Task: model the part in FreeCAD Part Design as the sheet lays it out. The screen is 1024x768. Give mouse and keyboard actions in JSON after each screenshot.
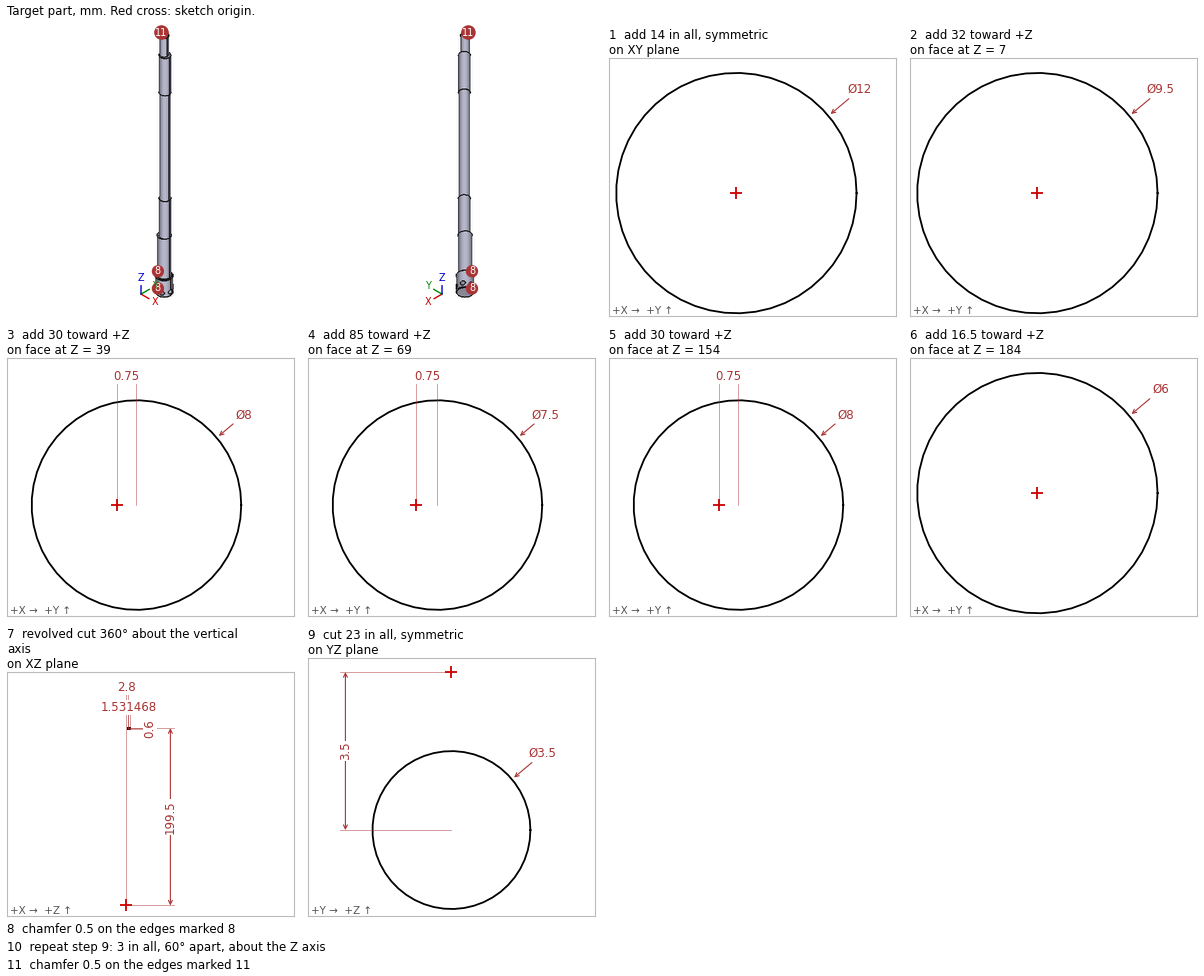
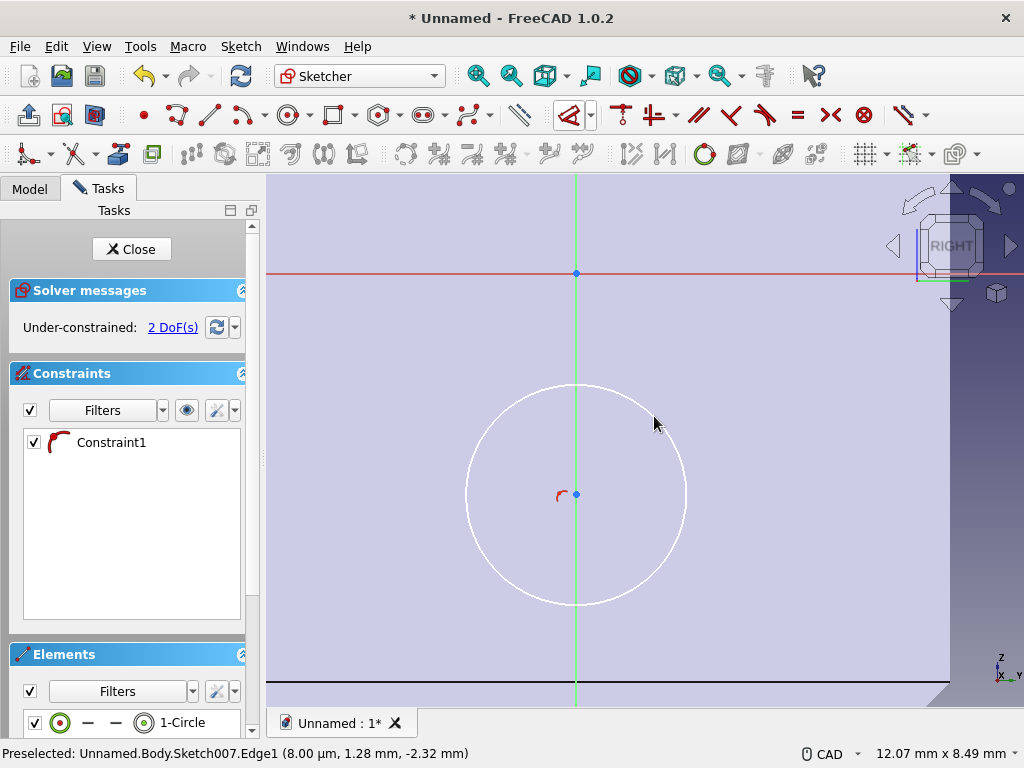
{"action": "left_click", "coordinate": [654, 417]}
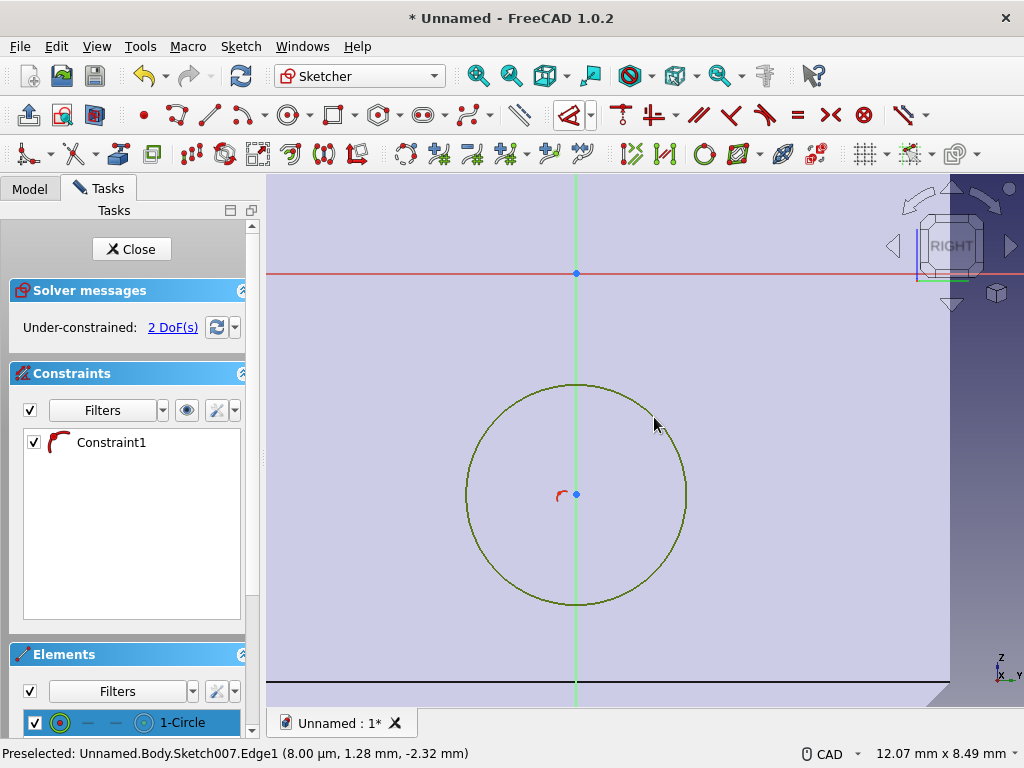
{"action": "left_click", "coordinate": [590, 116]}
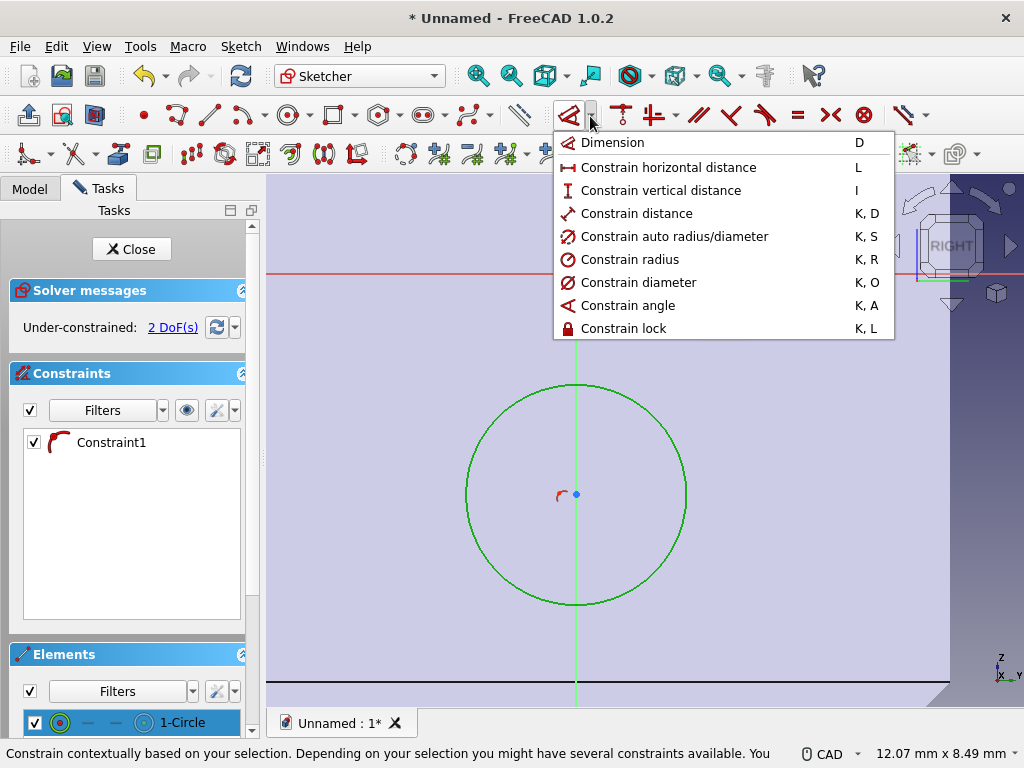
{"action": "left_click", "coordinate": [724, 282]}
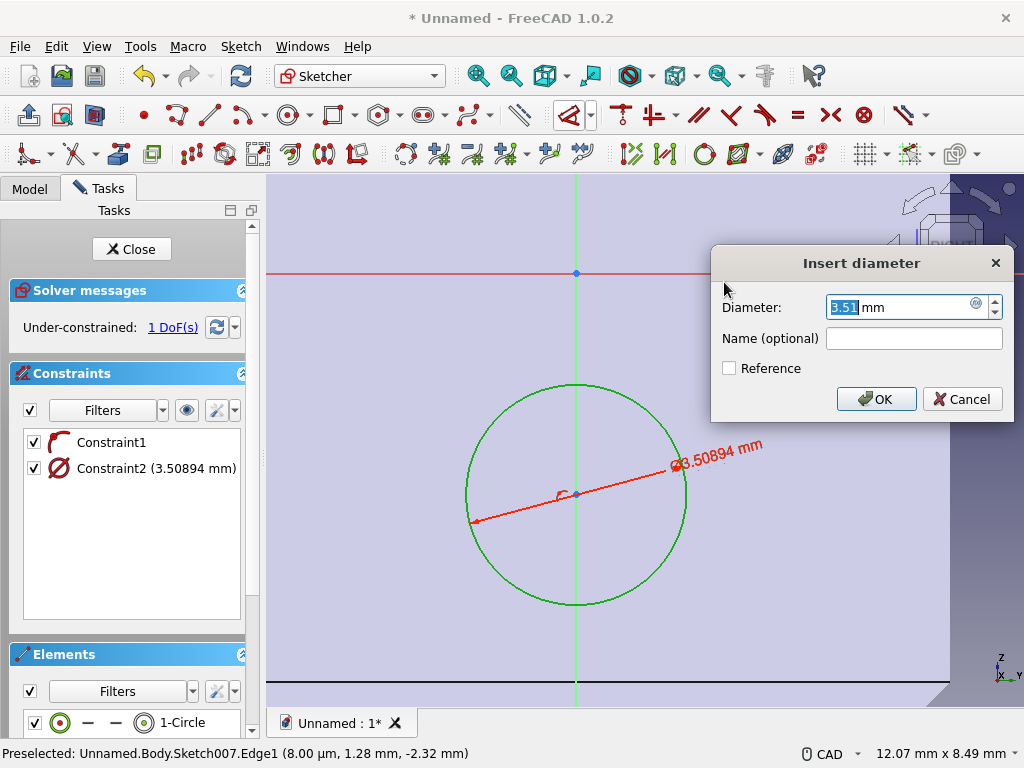
{"action": "type", "text": "3.5"}
{"action": "key", "text": "Return"}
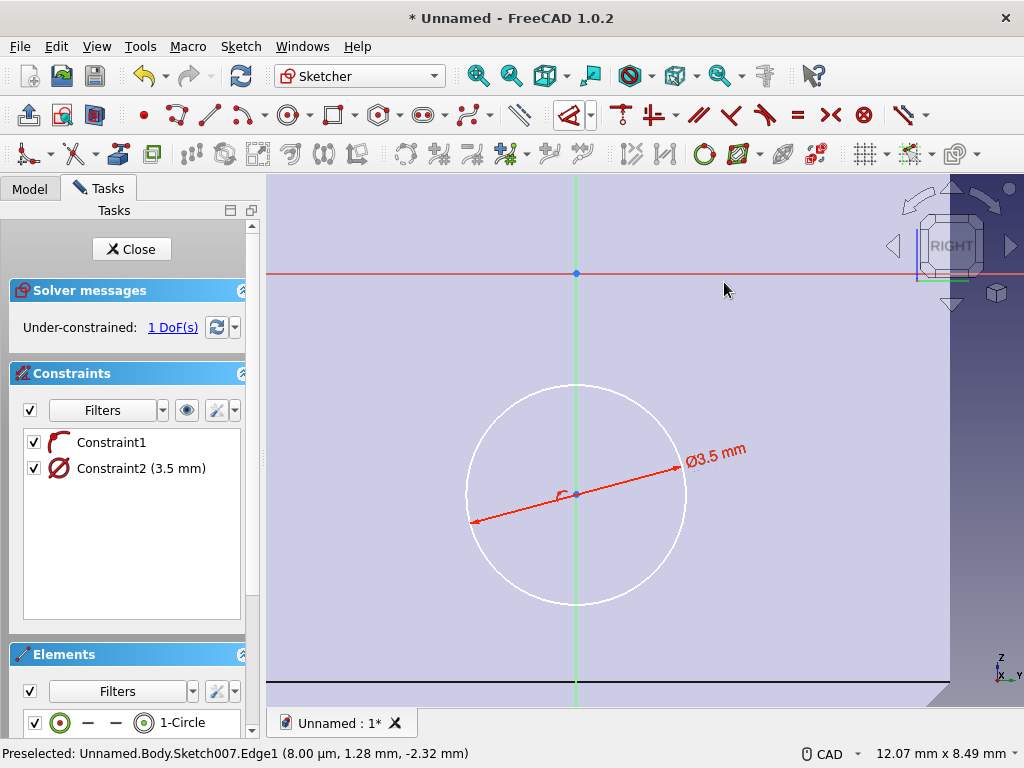
{"action": "left_click", "coordinate": [576, 495]}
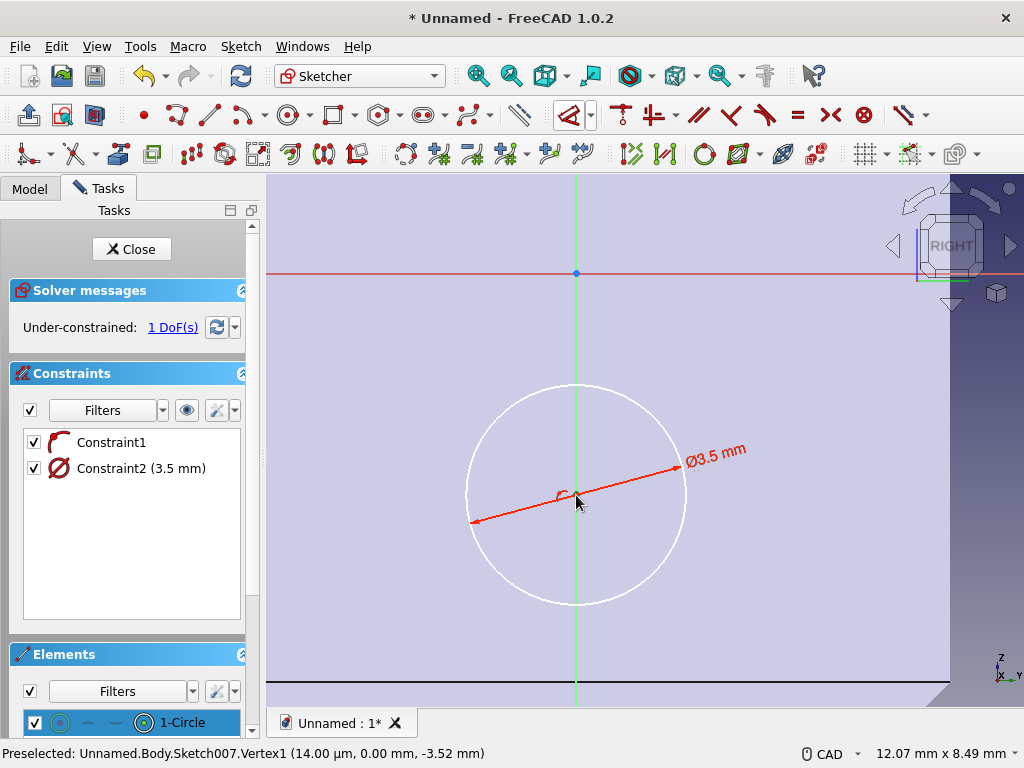
{"action": "key", "text": "i"}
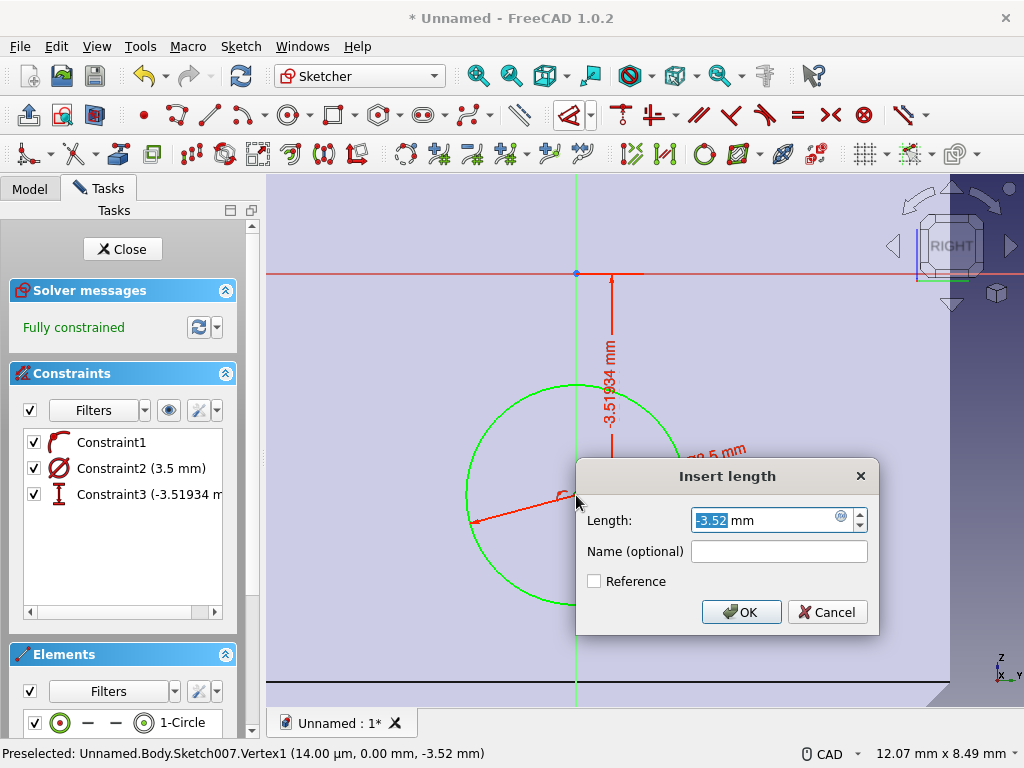
{"action": "type", "text": "-3.5"}
{"action": "key", "text": "Return"}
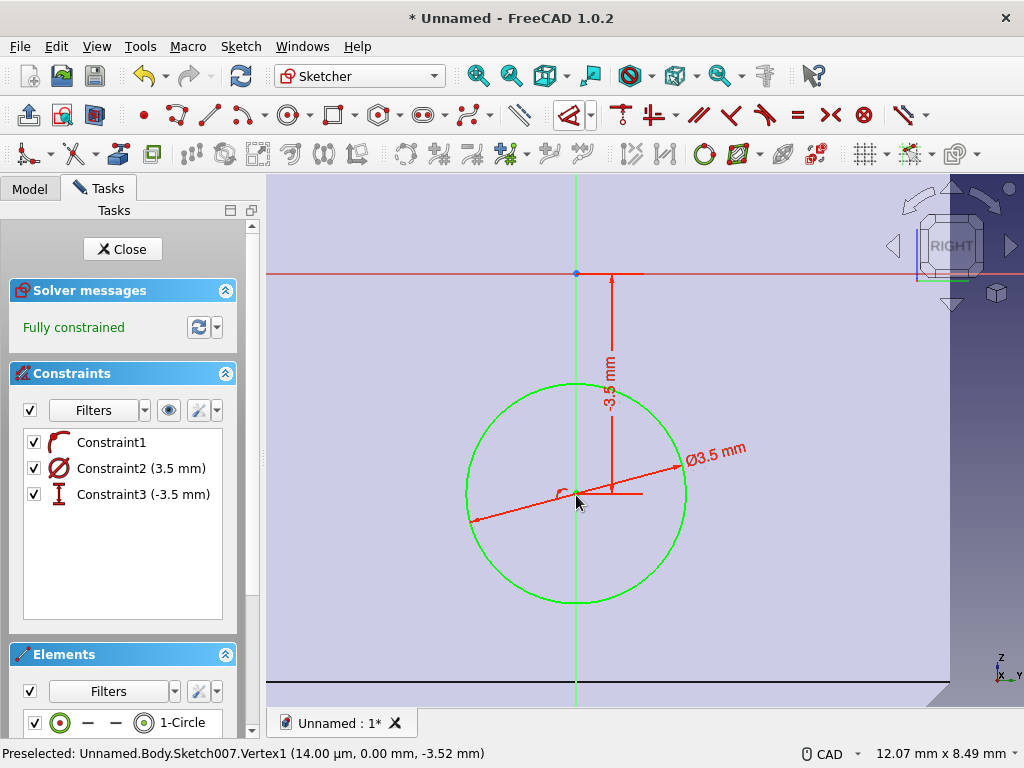
{"action": "left_click", "coordinate": [123, 249]}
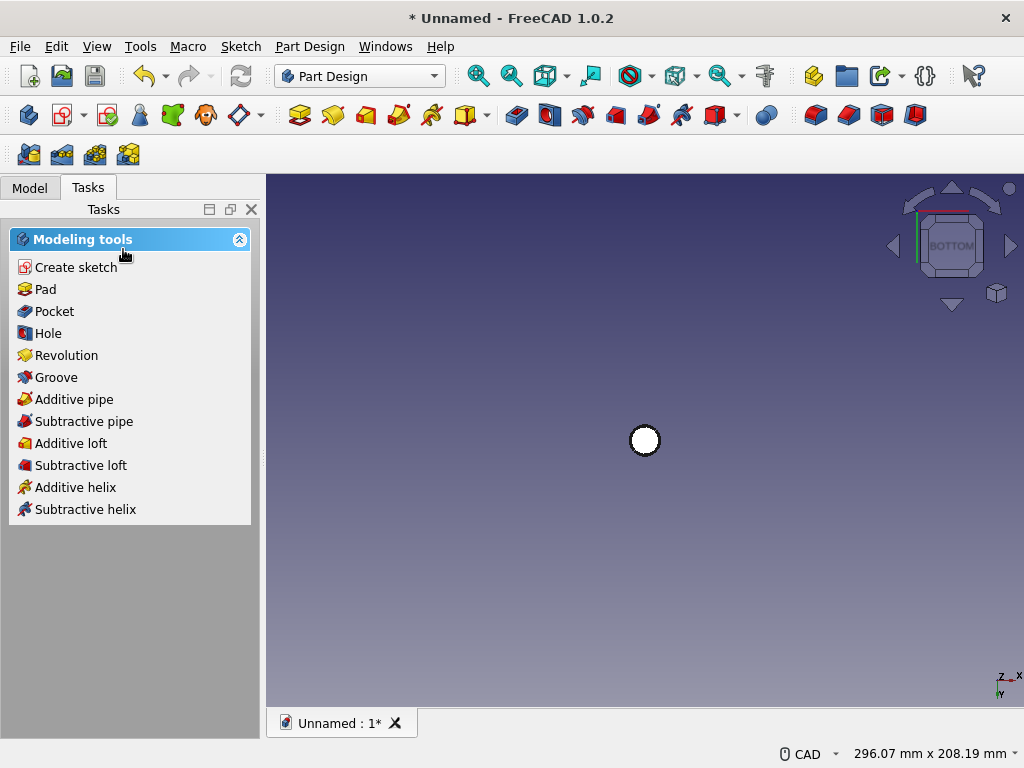
{"action": "left_click", "coordinate": [517, 116]}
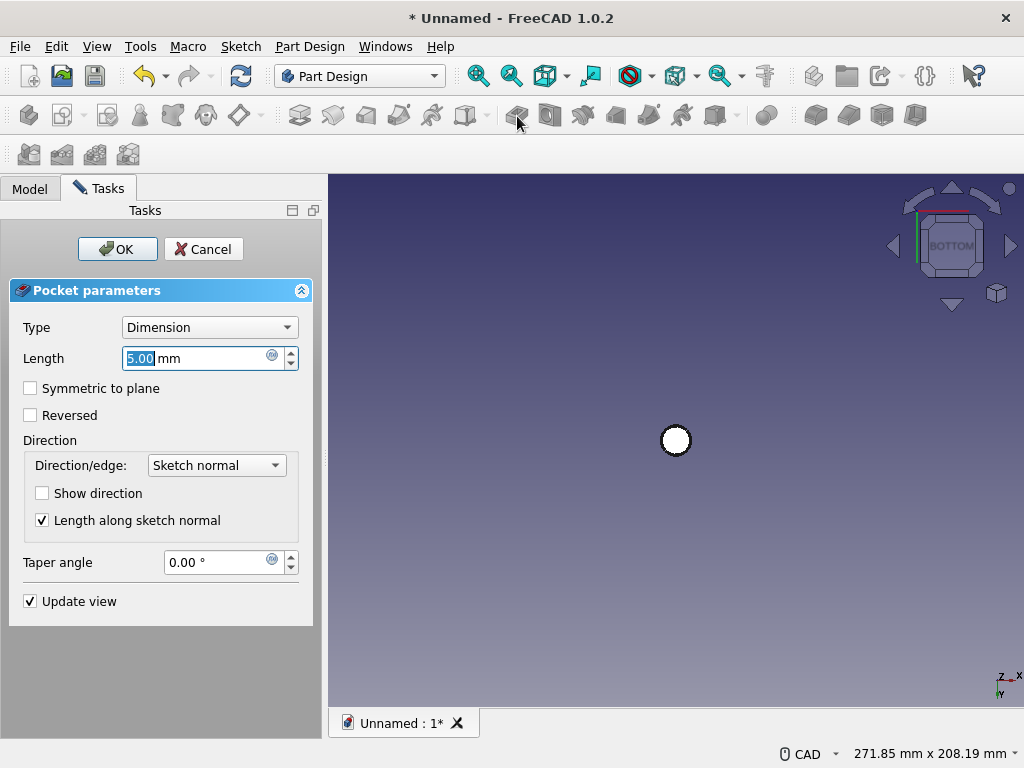
{"action": "type", "text": "23"}
{"action": "key", "text": "Tab"}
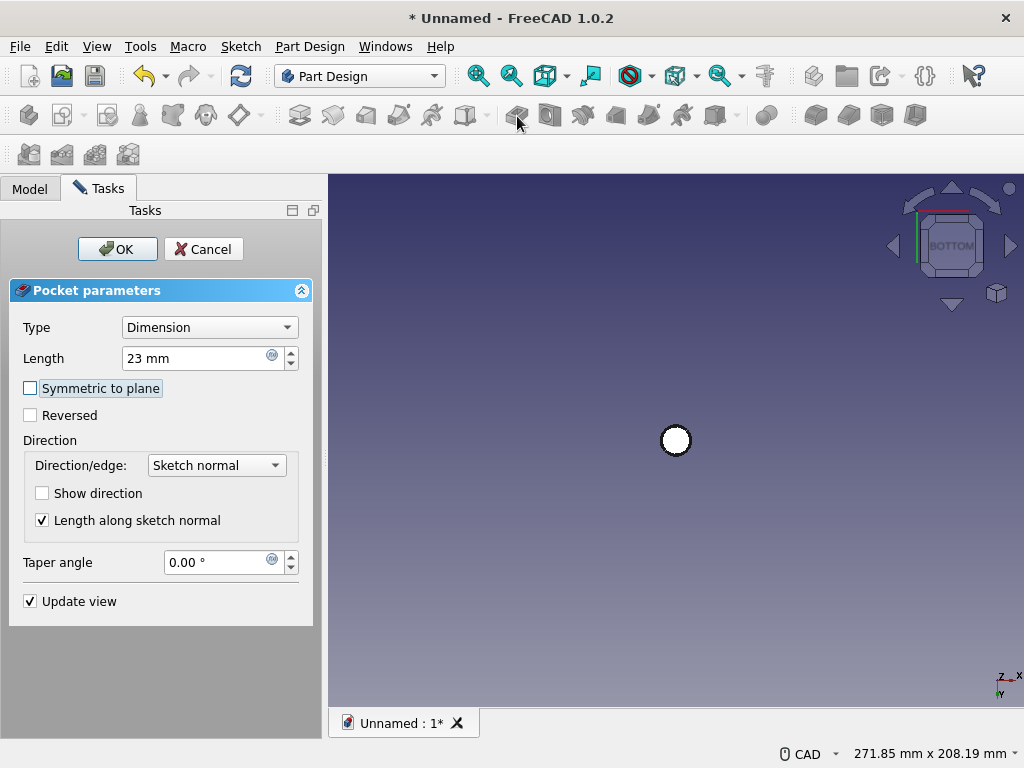
{"action": "left_click", "coordinate": [31, 388]}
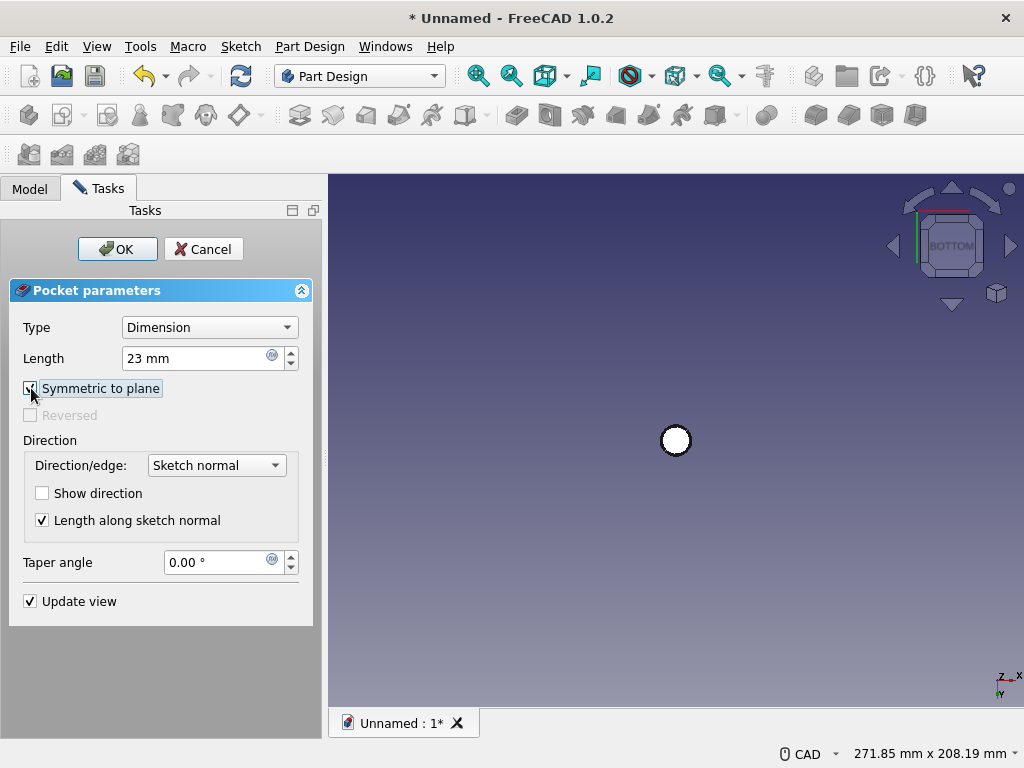
{"action": "left_click", "coordinate": [118, 249]}